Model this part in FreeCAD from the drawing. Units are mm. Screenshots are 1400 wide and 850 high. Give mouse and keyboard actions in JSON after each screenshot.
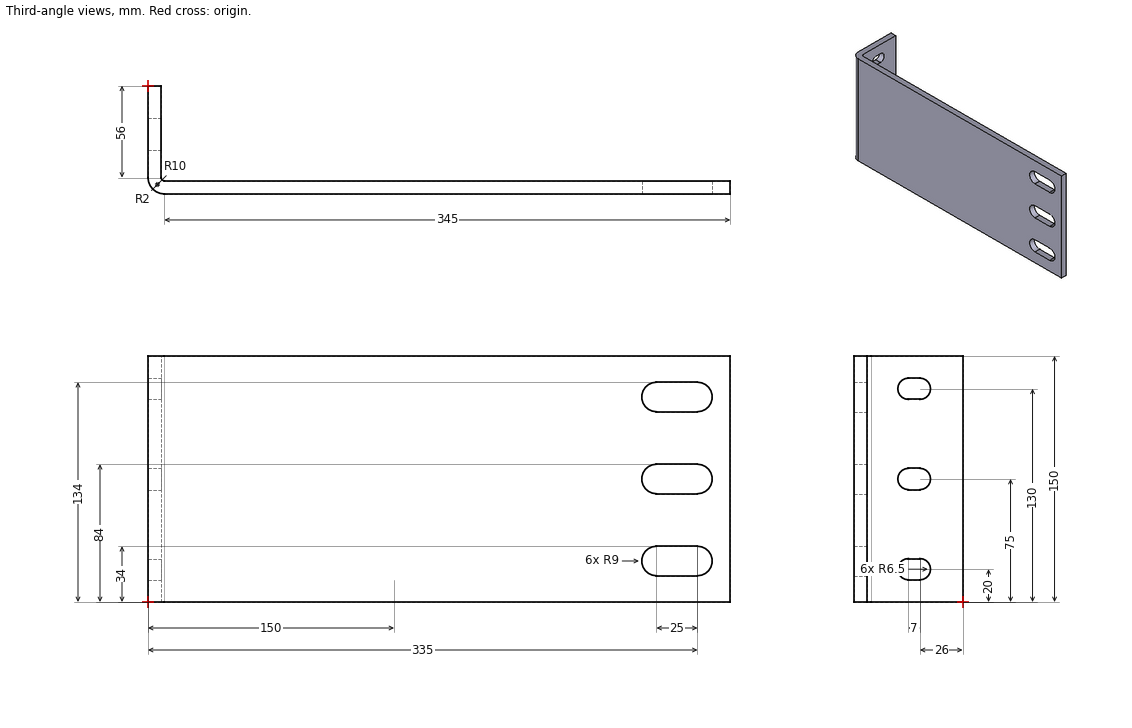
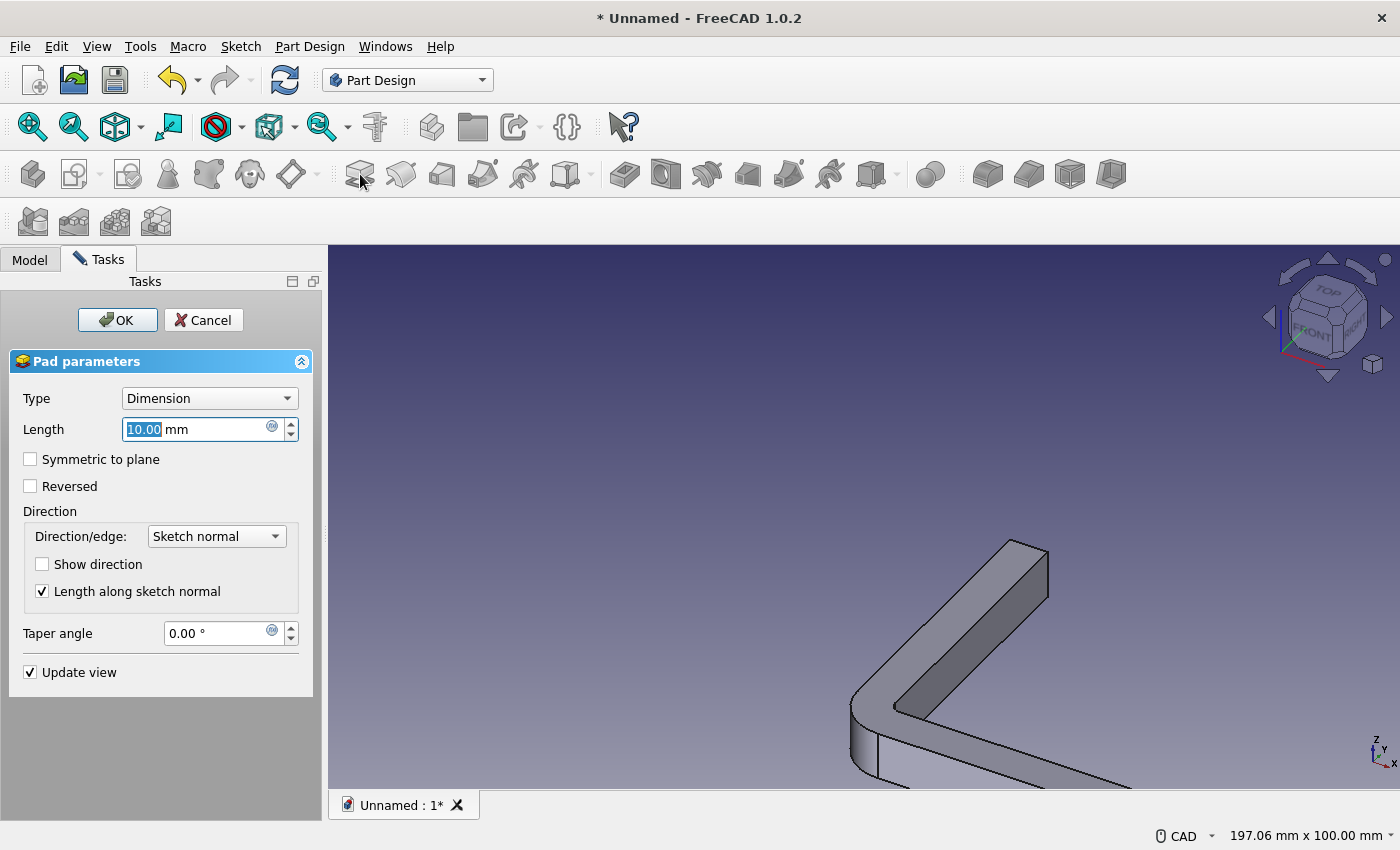
{"action": "type", "text": "150"}
{"action": "key", "text": "Tab"}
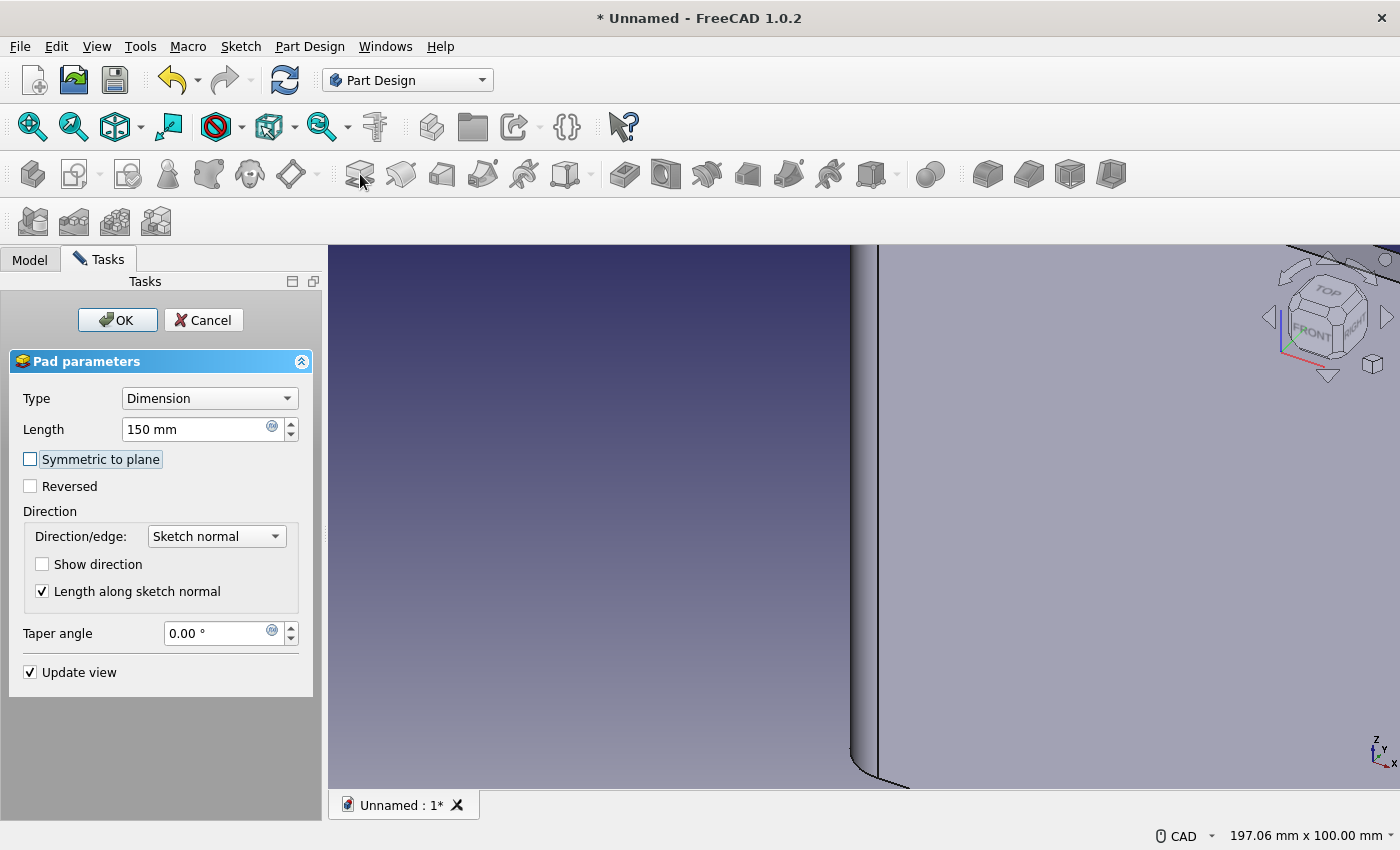
{"action": "left_click", "coordinate": [118, 320]}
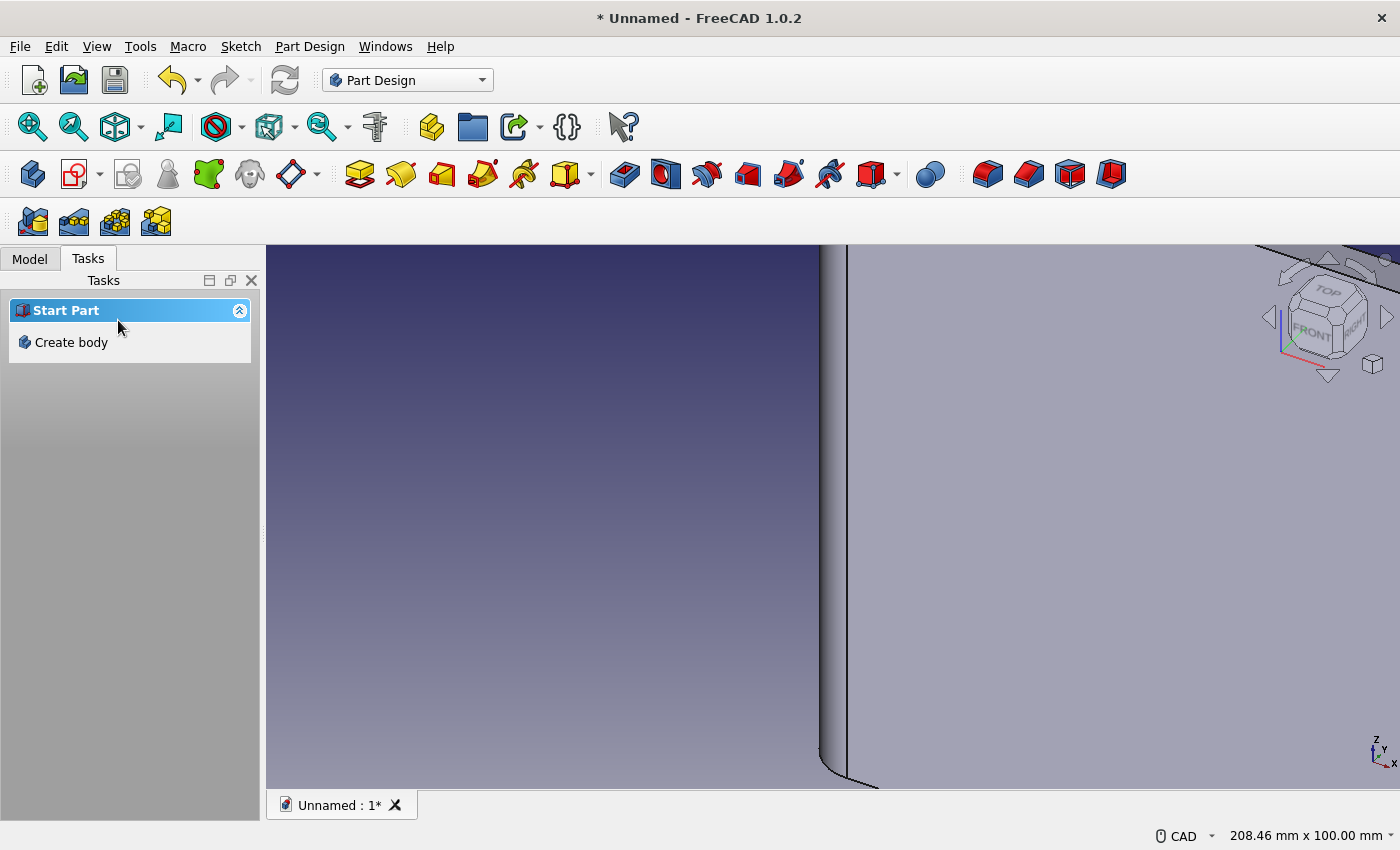
{"action": "left_click", "coordinate": [33, 128]}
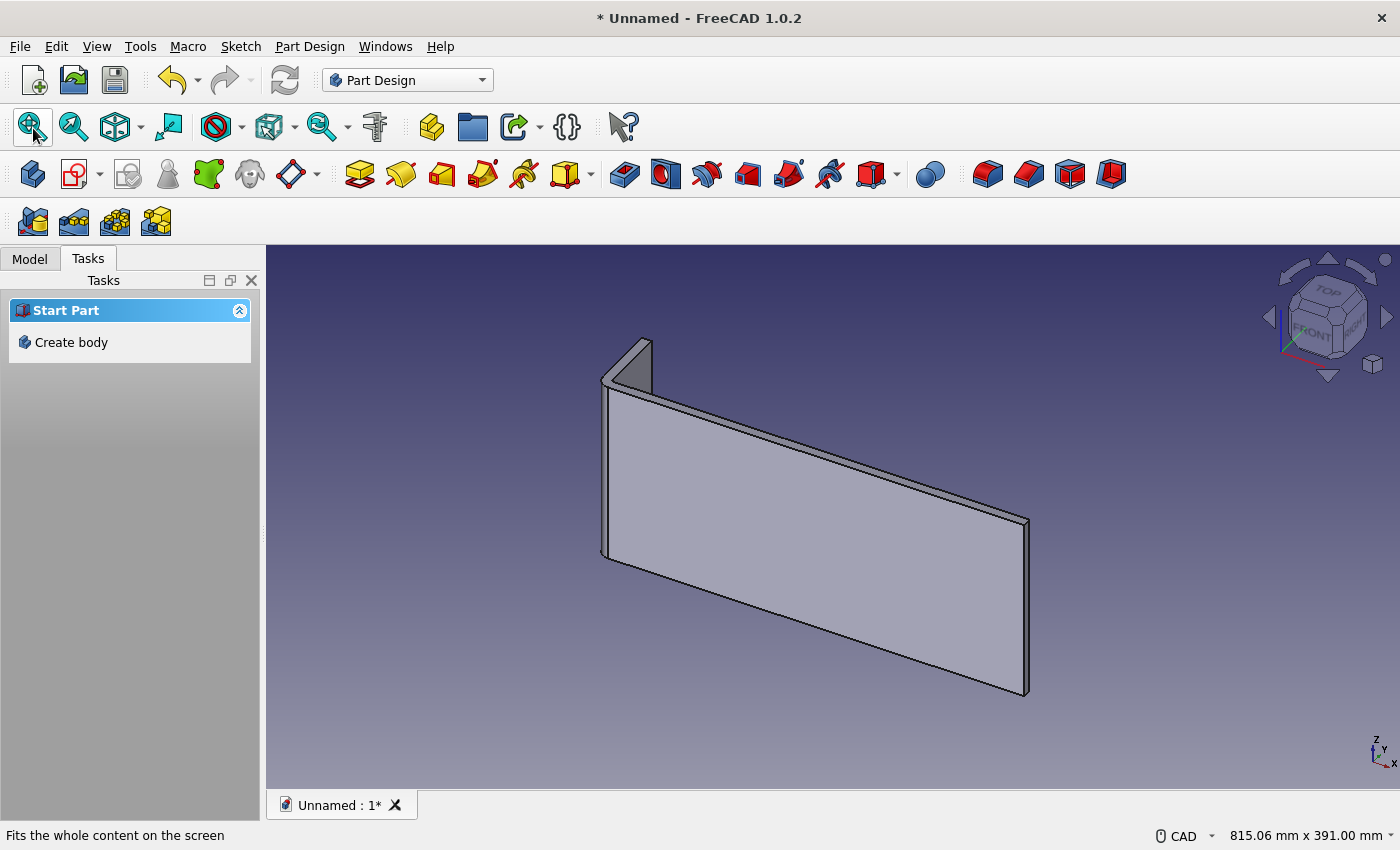
{"action": "key", "text": "6"}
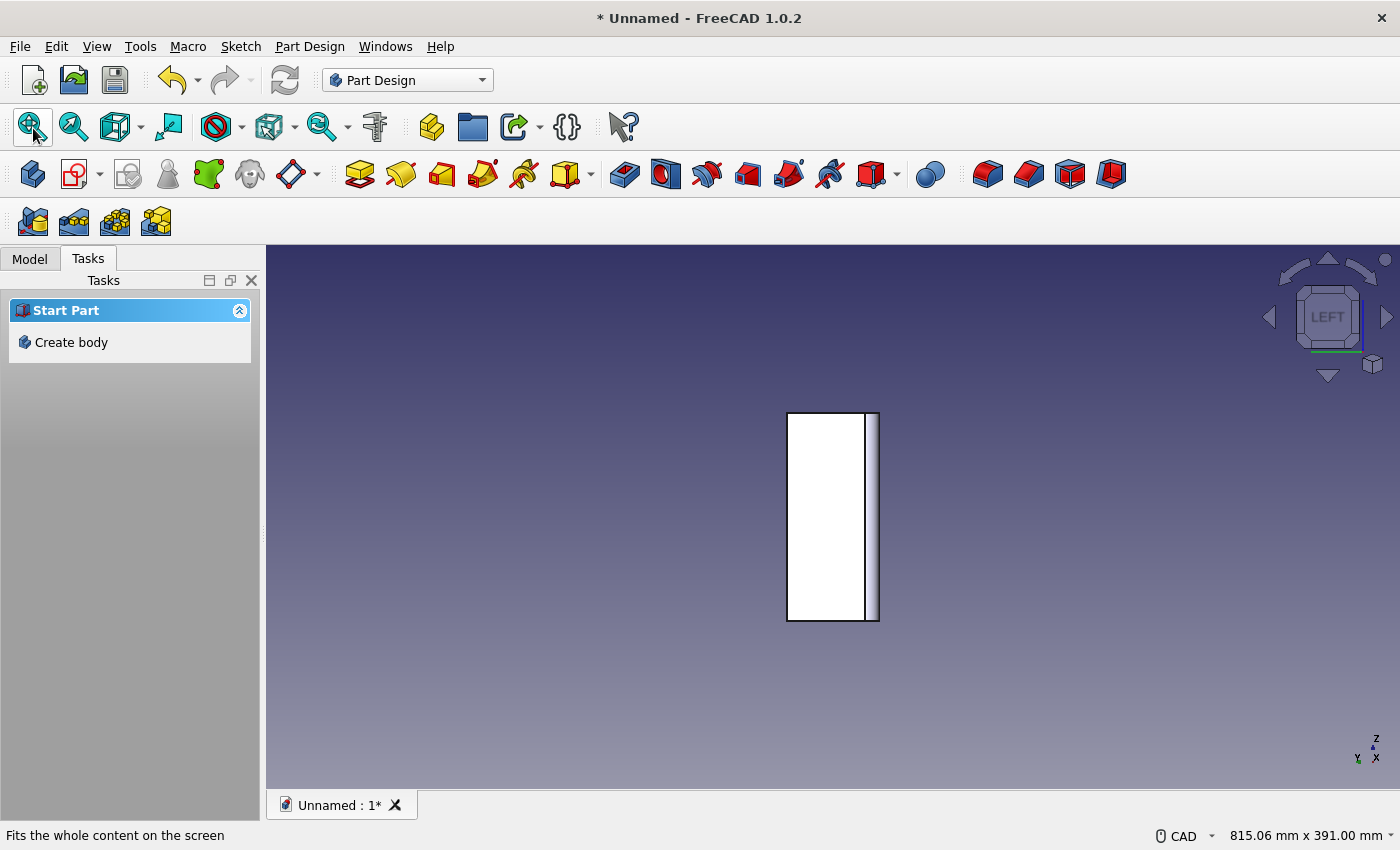
{"action": "left_click", "coordinate": [33, 128]}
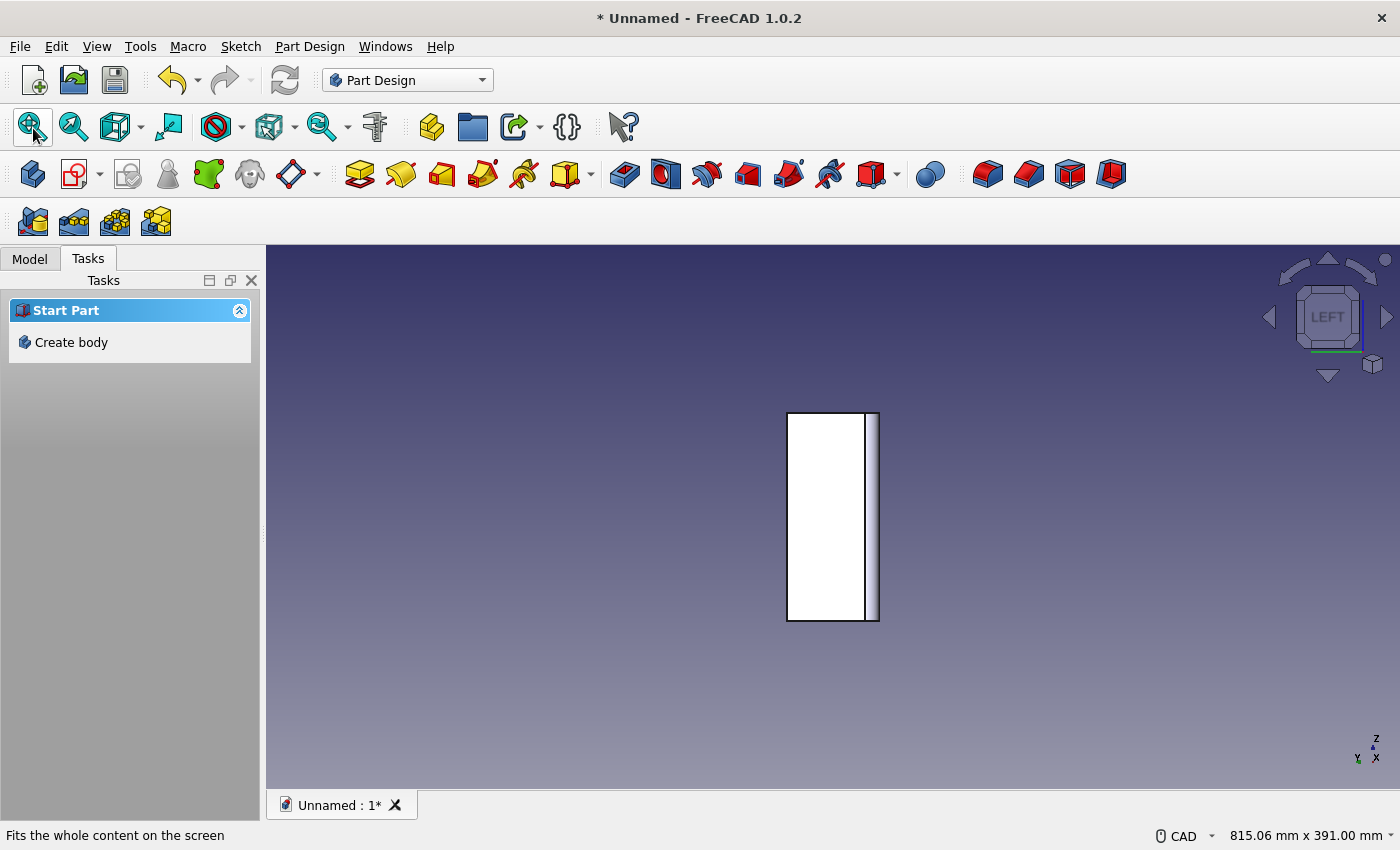
{"action": "left_click", "coordinate": [826, 456]}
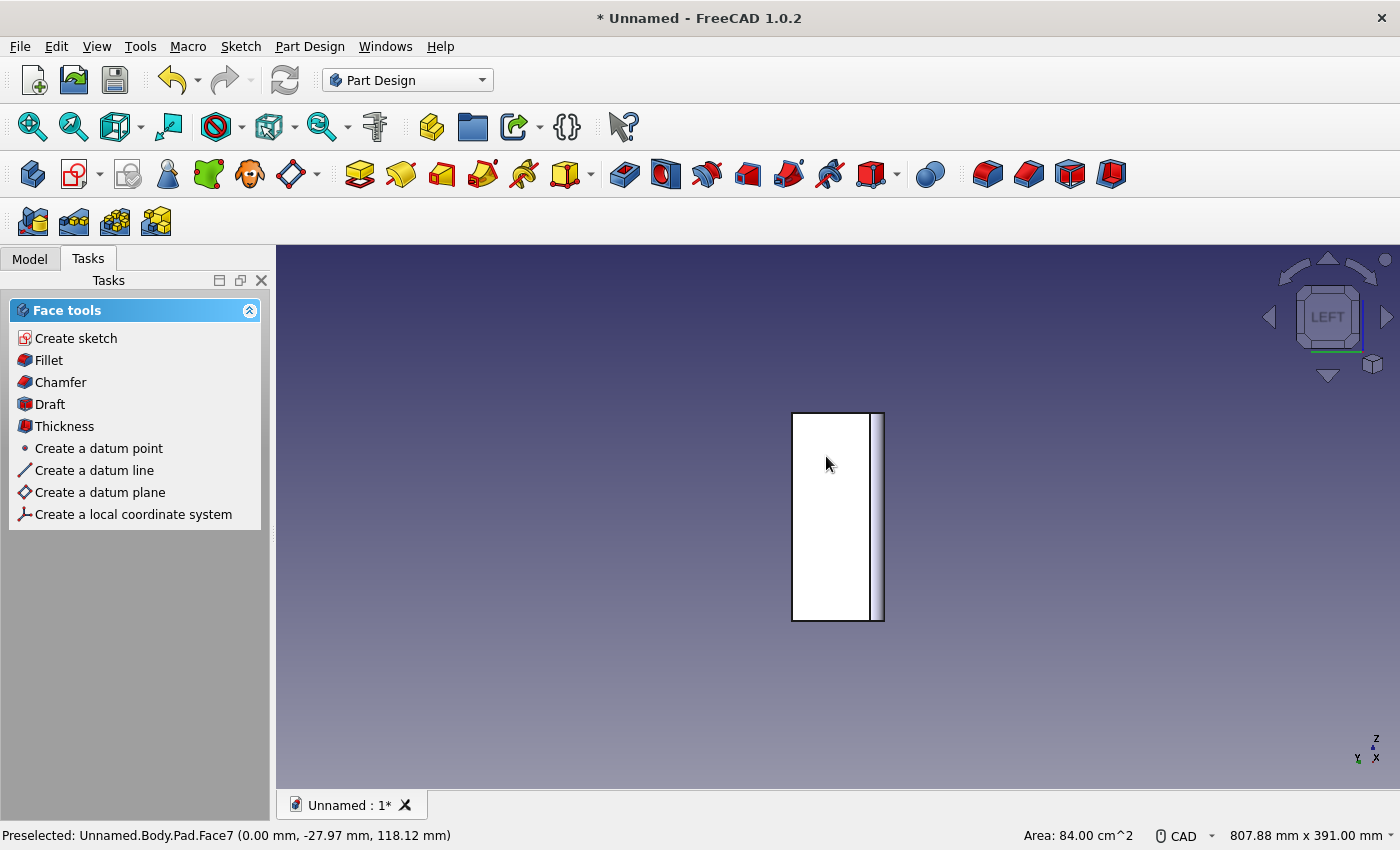
{"action": "left_click", "coordinate": [74, 174]}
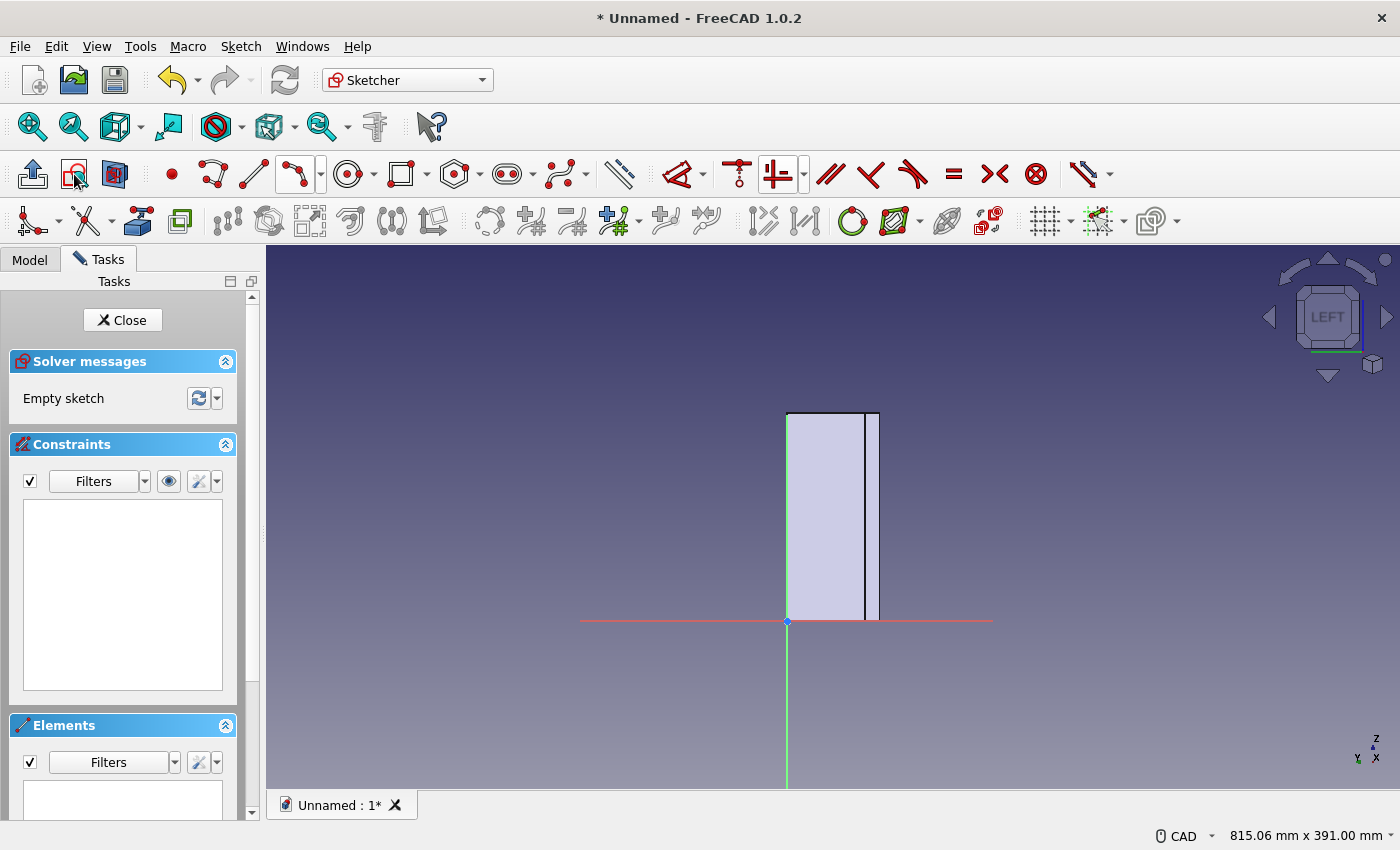
{"action": "scroll", "coordinate": [875, 538], "scroll_direction": "up", "scroll_amount": 3}